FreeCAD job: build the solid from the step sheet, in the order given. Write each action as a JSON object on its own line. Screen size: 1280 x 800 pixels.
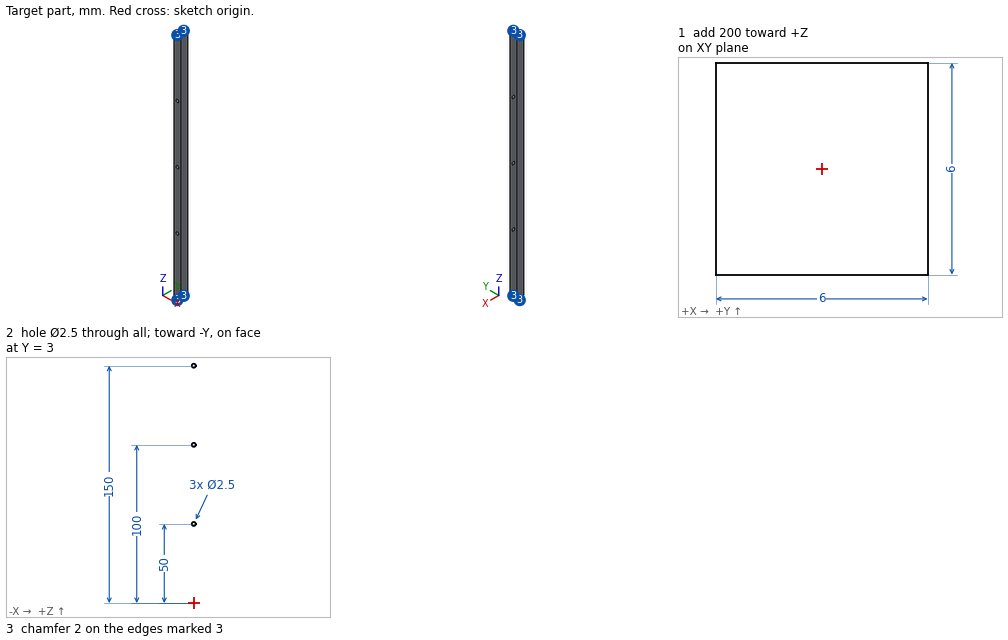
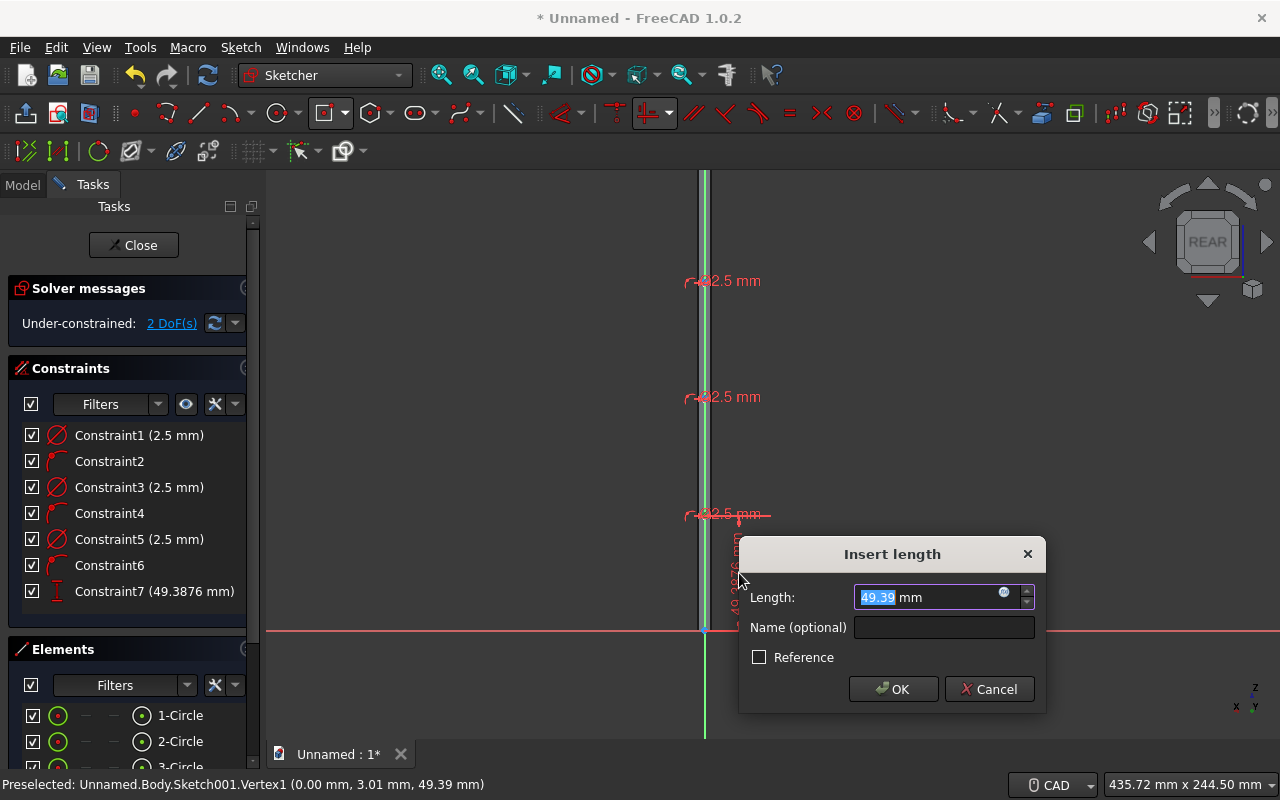
{"action": "type", "text": "50"}
{"action": "key", "text": "Return"}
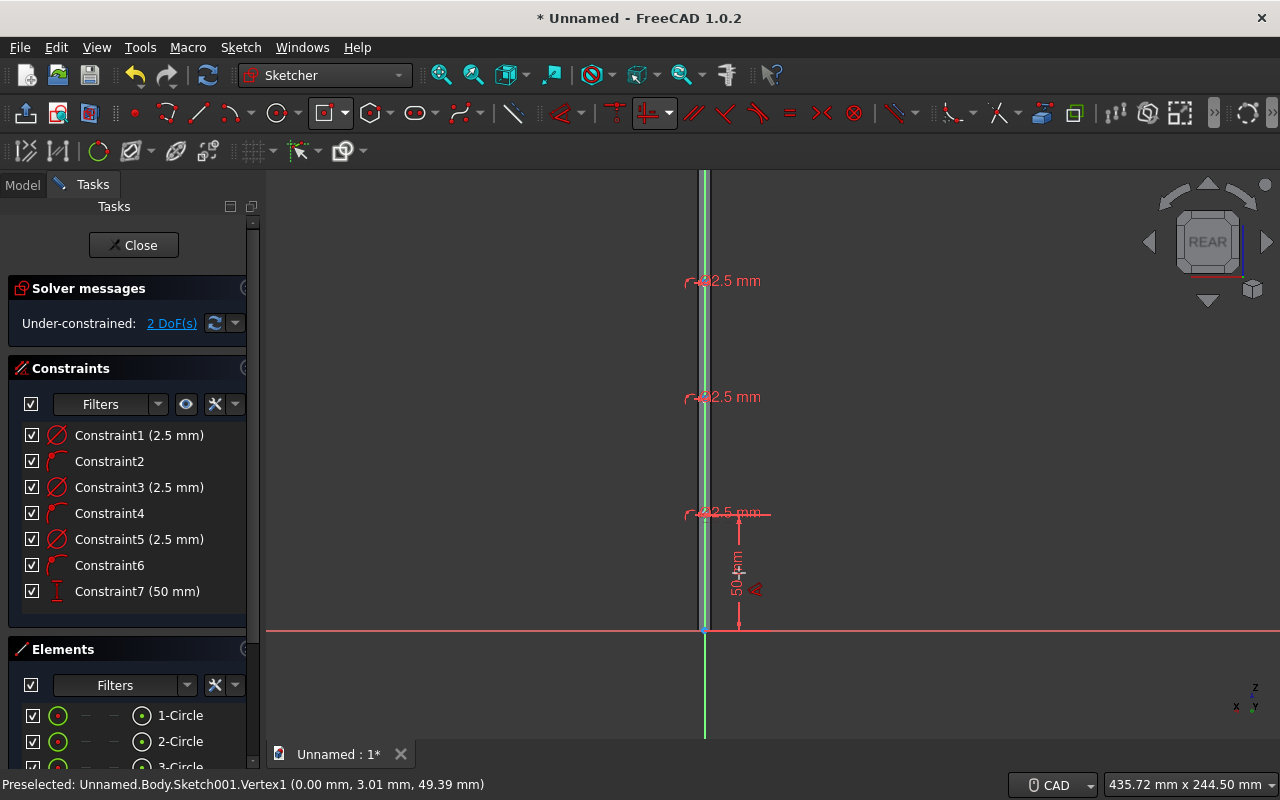
{"action": "left_click", "coordinate": [705, 399]}
{"action": "left_click", "coordinate": [739, 515]}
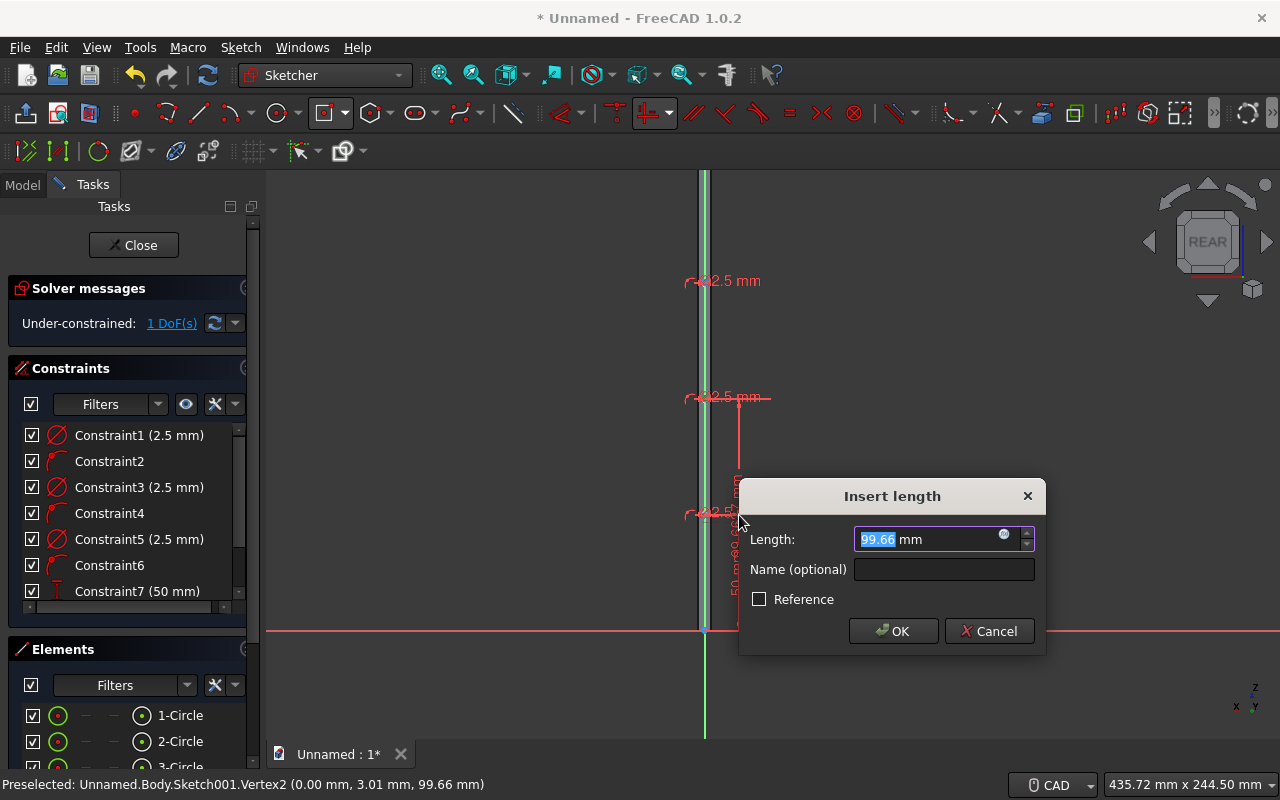
{"action": "type", "text": "100"}
{"action": "key", "text": "Return"}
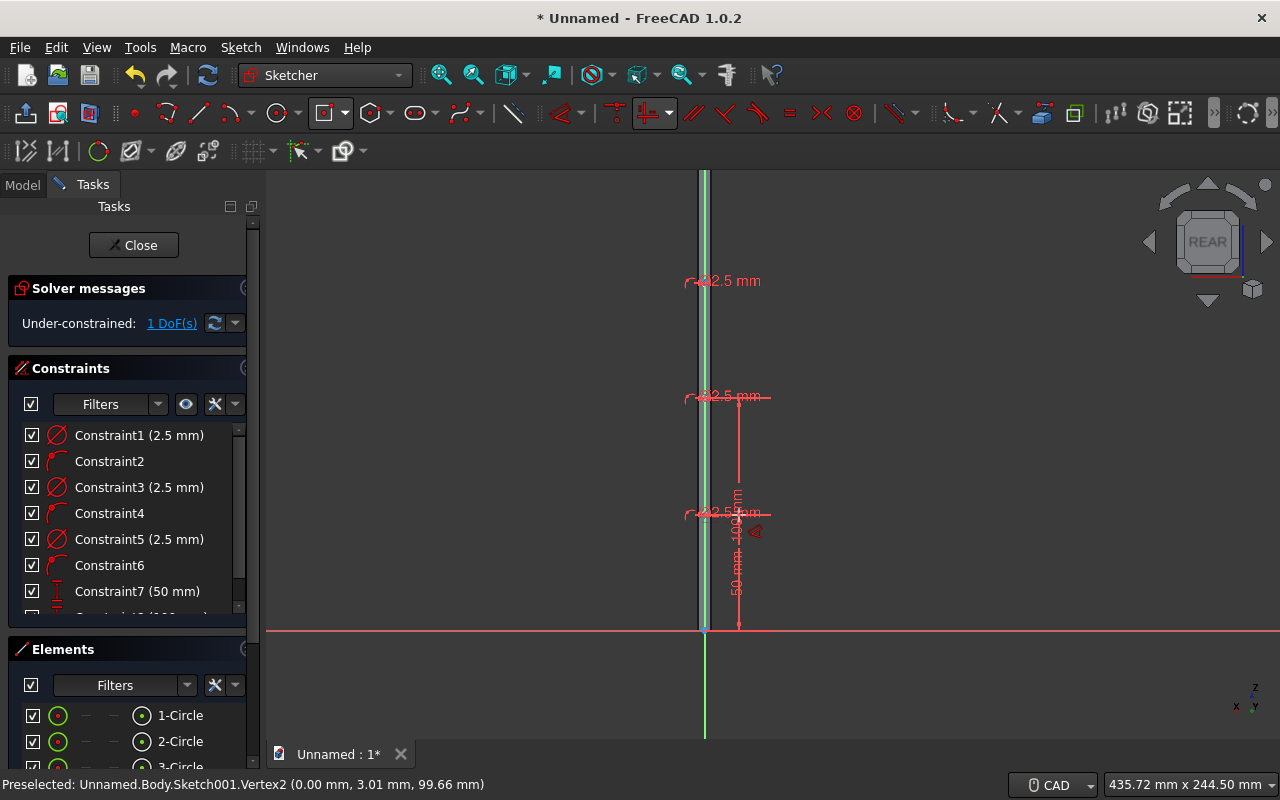
{"action": "left_click", "coordinate": [705, 283]}
{"action": "left_click", "coordinate": [739, 457]}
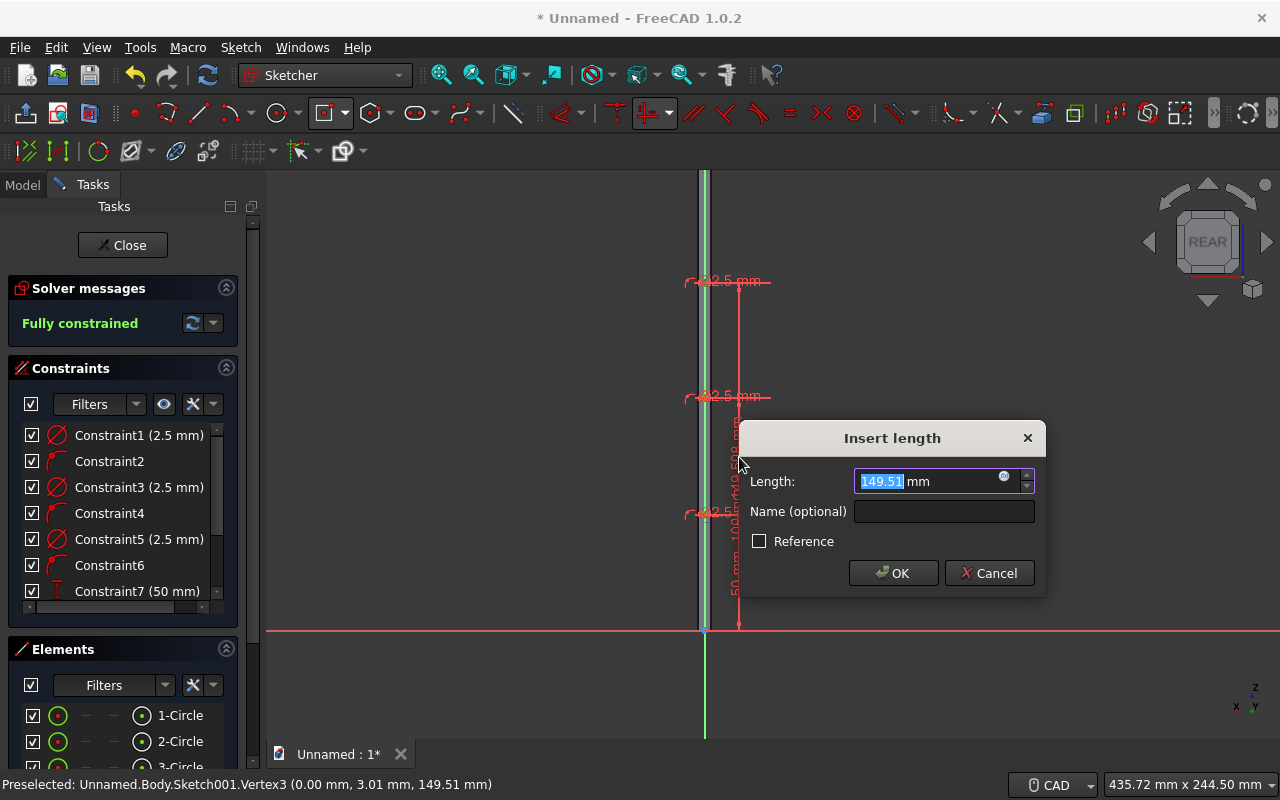
{"action": "type", "text": "150"}
{"action": "key", "text": "Return"}
{"action": "key", "text": "Escape"}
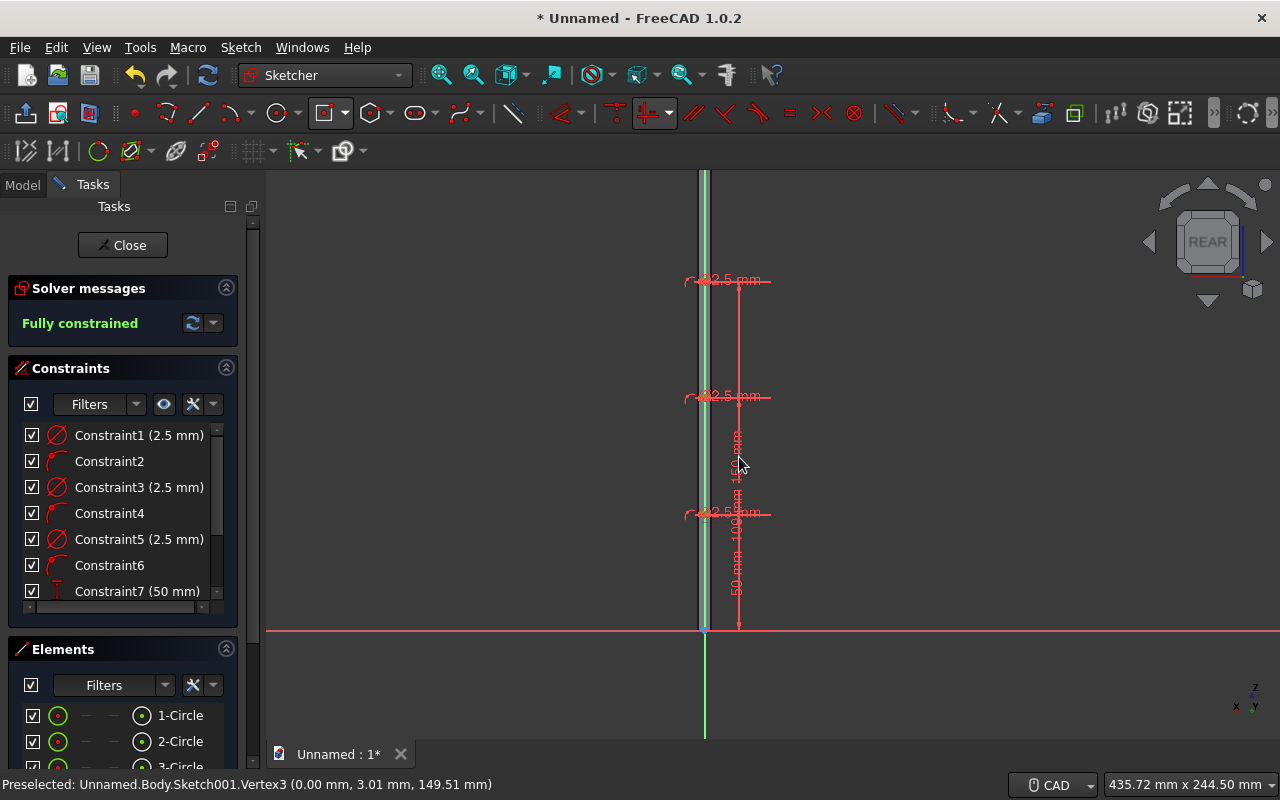
{"action": "left_click", "coordinate": [123, 245]}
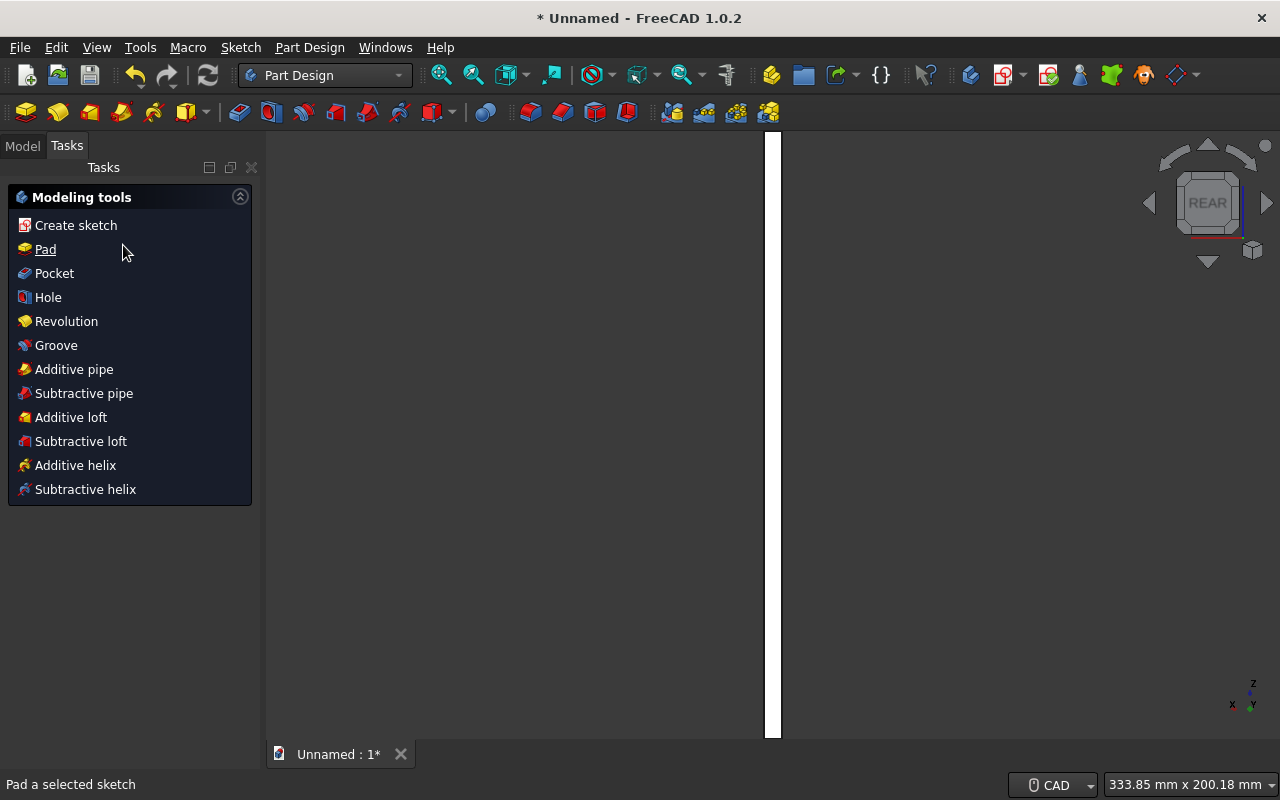
{"action": "left_click", "coordinate": [272, 112]}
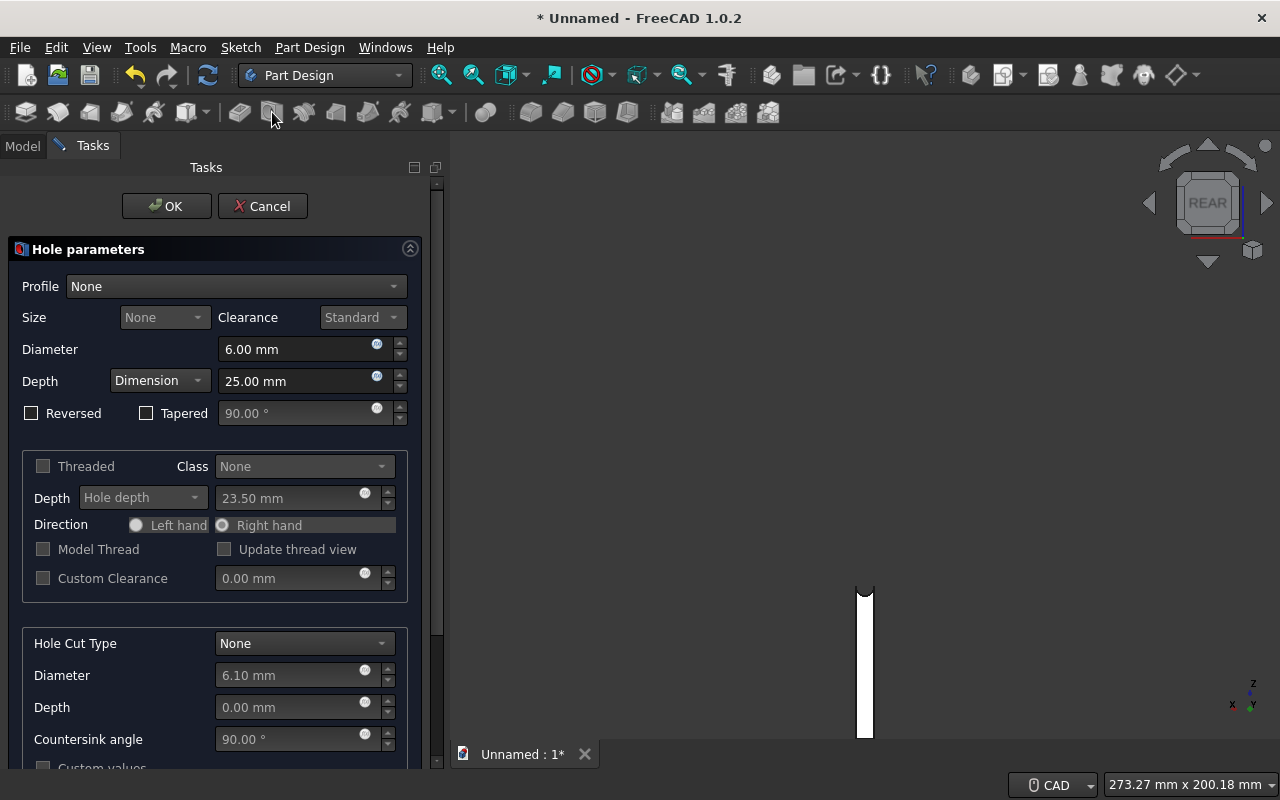
{"action": "triple_click", "coordinate": [305, 349]}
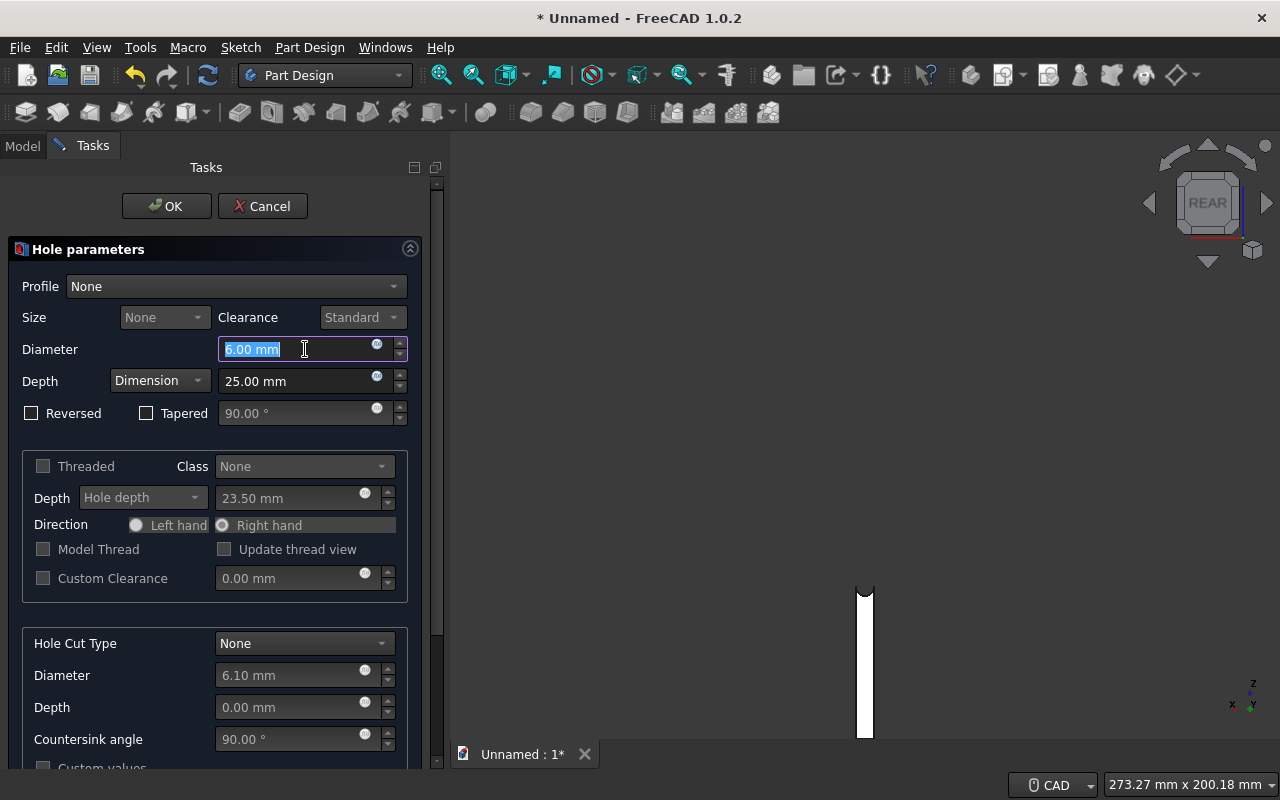
{"action": "type", "text": "2.5"}
{"action": "key", "text": "Tab"}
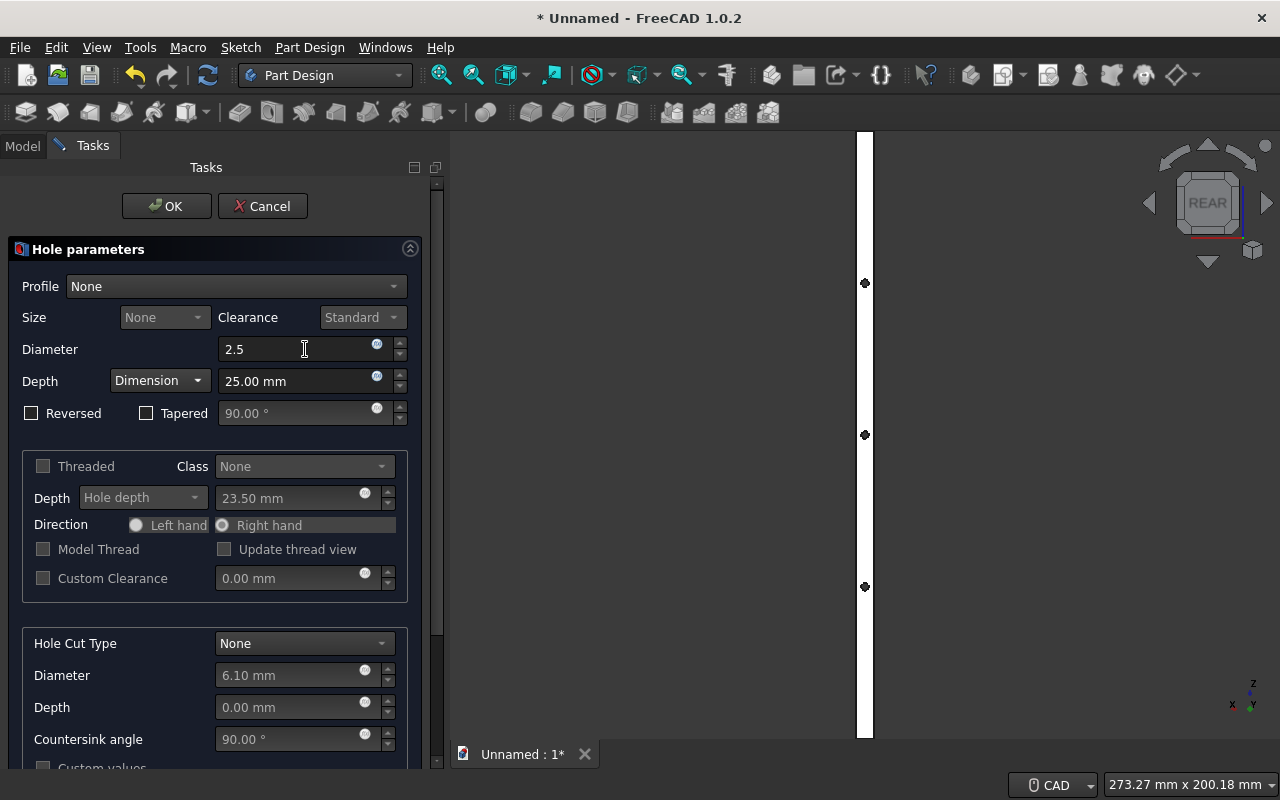
{"action": "left_click", "coordinate": [161, 380]}